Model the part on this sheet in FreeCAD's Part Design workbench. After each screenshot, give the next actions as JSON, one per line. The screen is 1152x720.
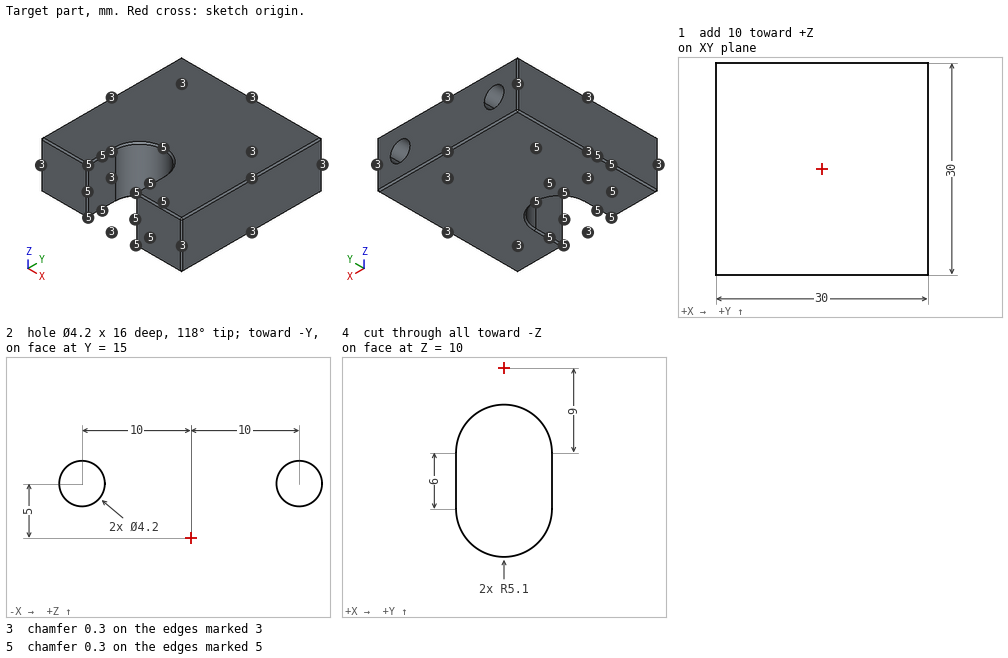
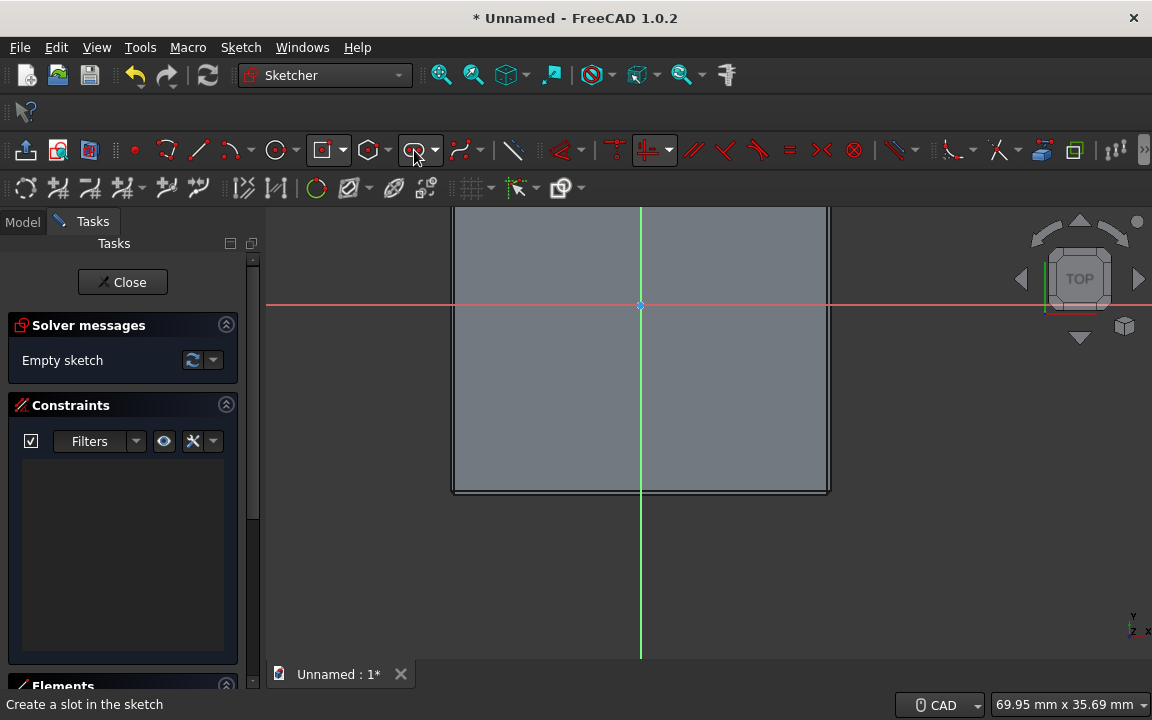
{"action": "left_click", "coordinate": [641, 495]}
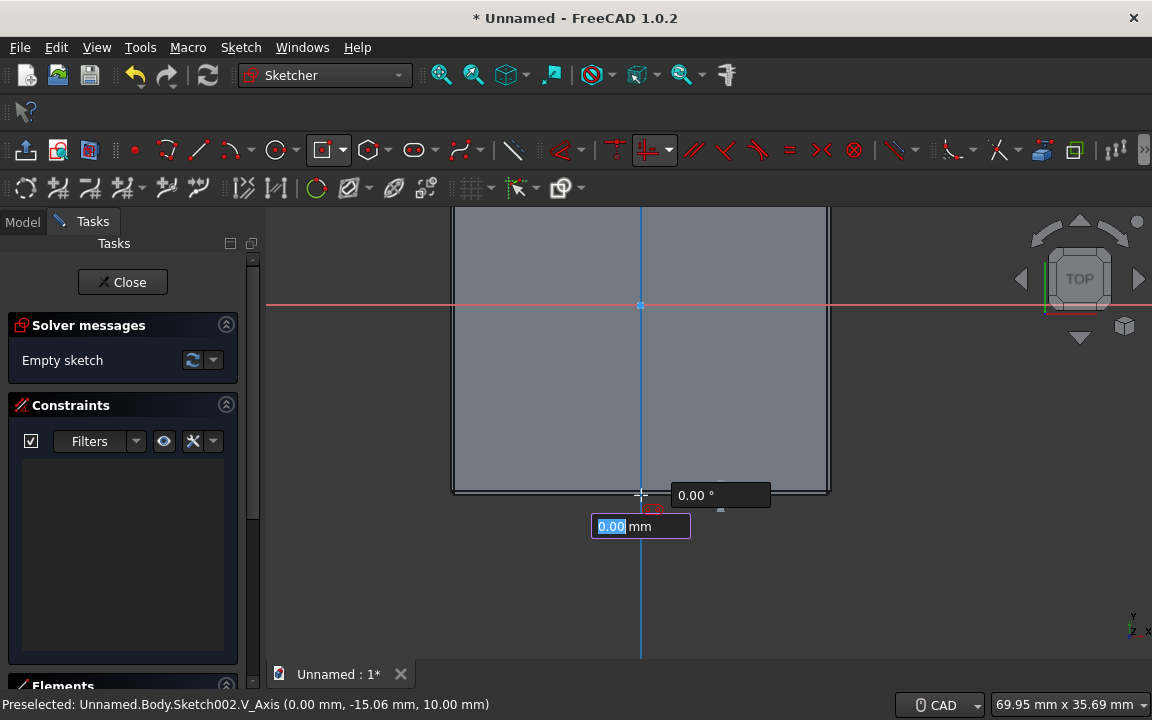
{"action": "left_click", "coordinate": [650, 419]}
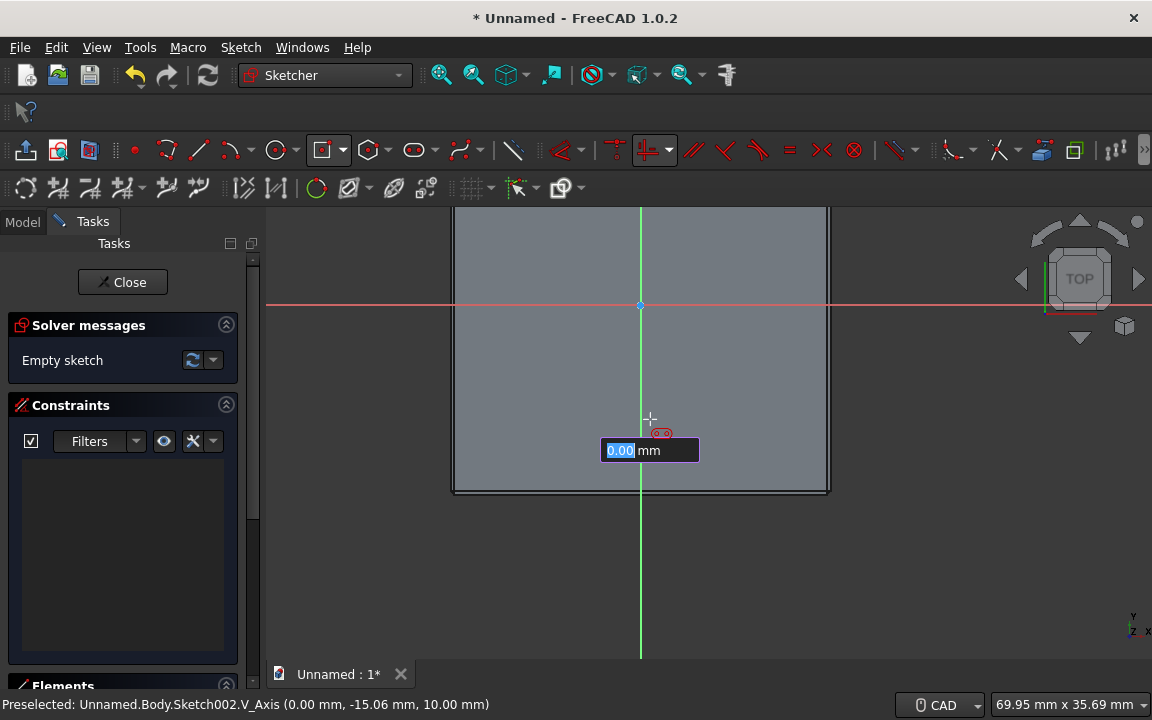
{"action": "left_click", "coordinate": [576, 457]}
{"action": "key", "text": "Escape"}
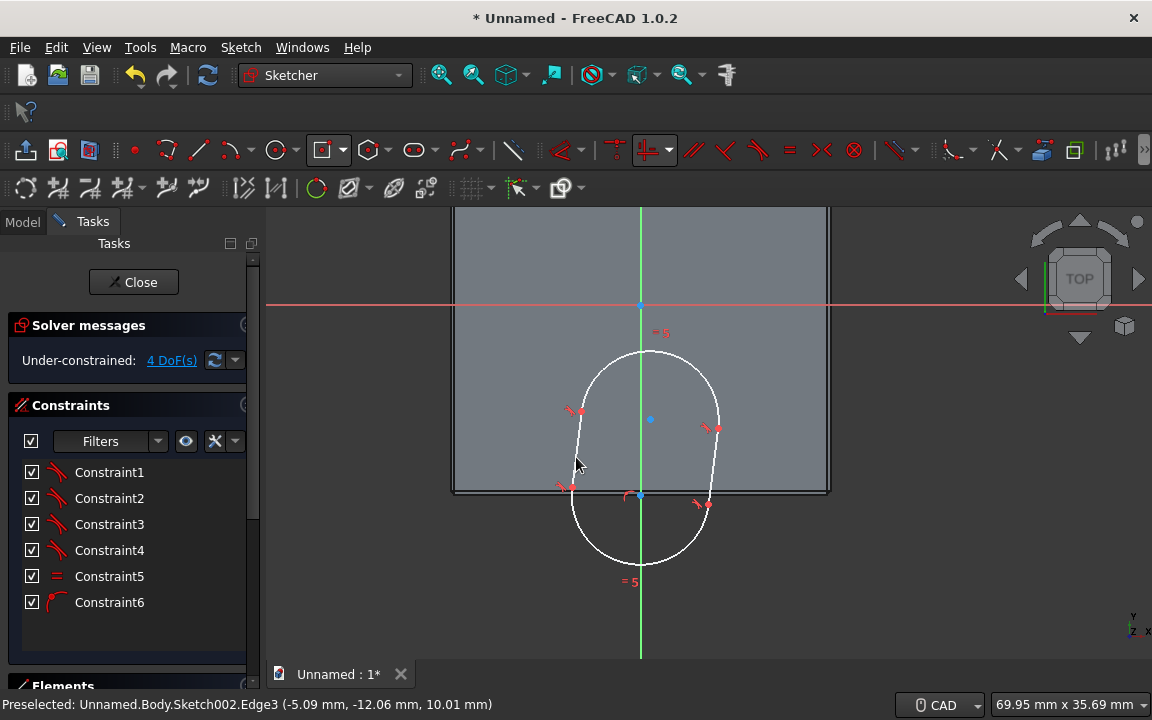
{"action": "left_click", "coordinate": [575, 465]}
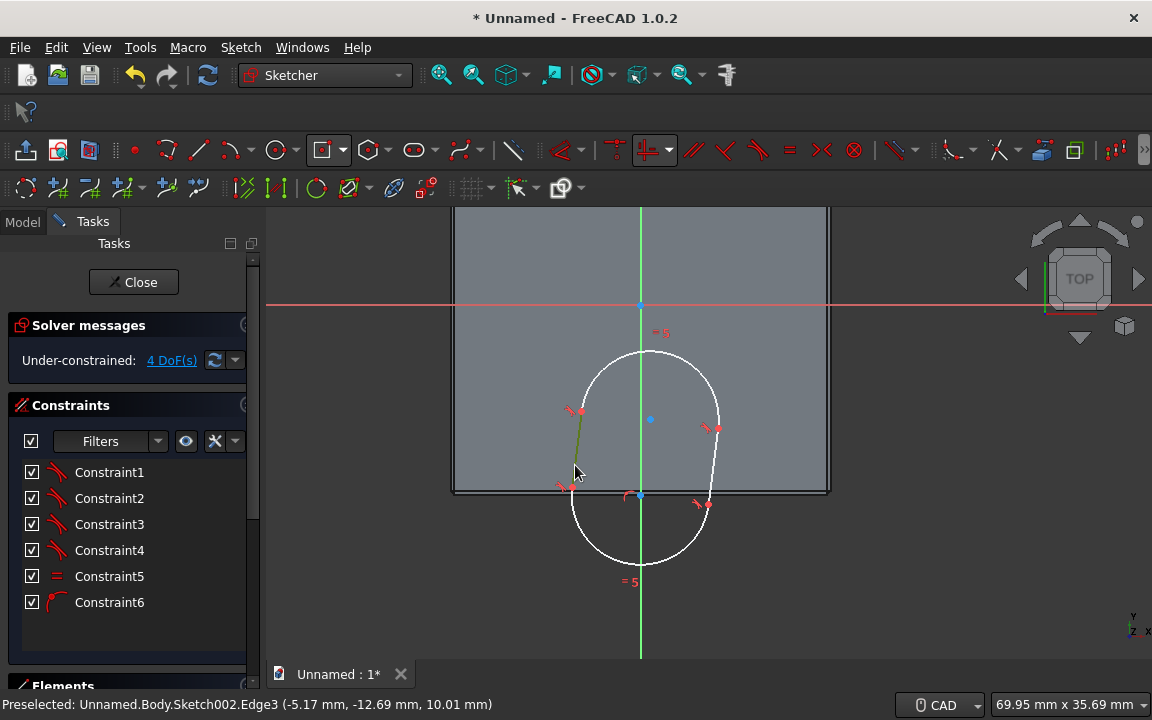
{"action": "left_click", "coordinate": [672, 150]}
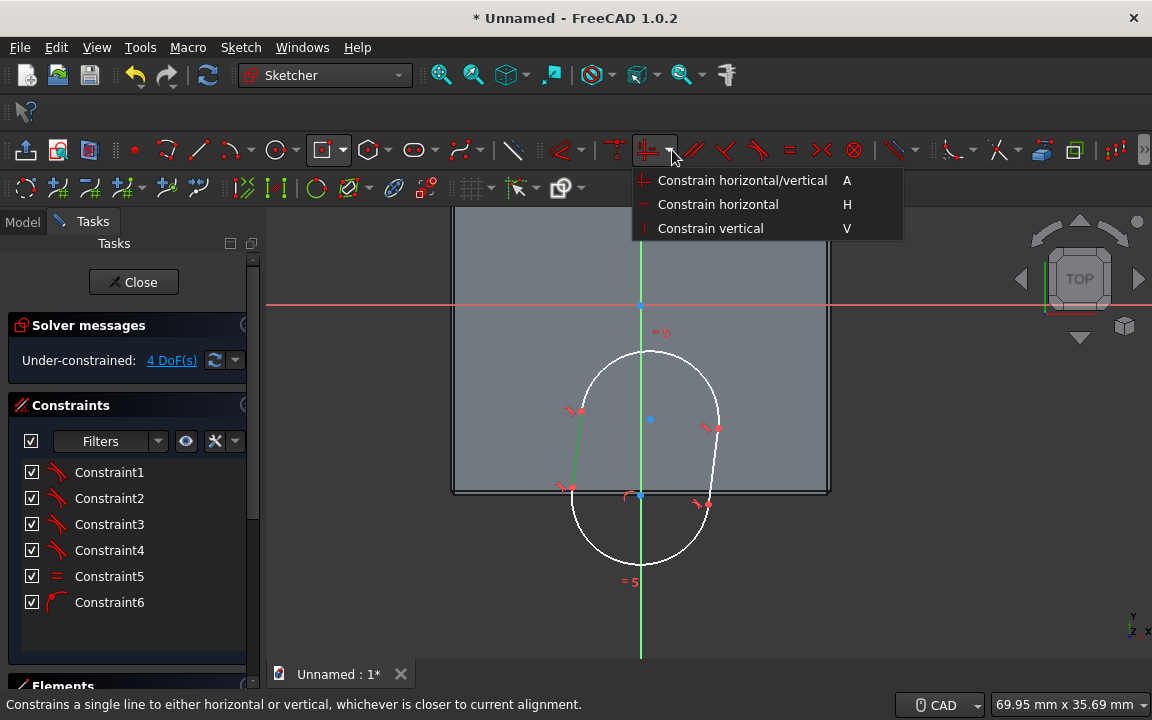
{"action": "left_click", "coordinate": [768, 228]}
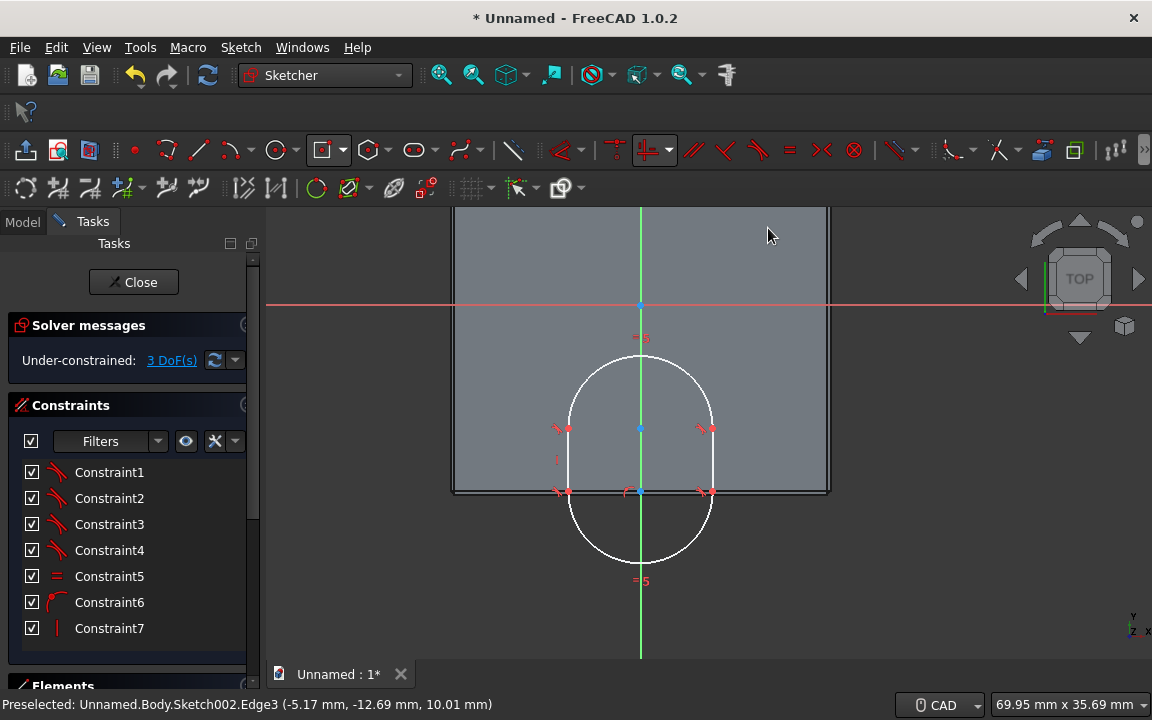
{"action": "left_click", "coordinate": [560, 150]}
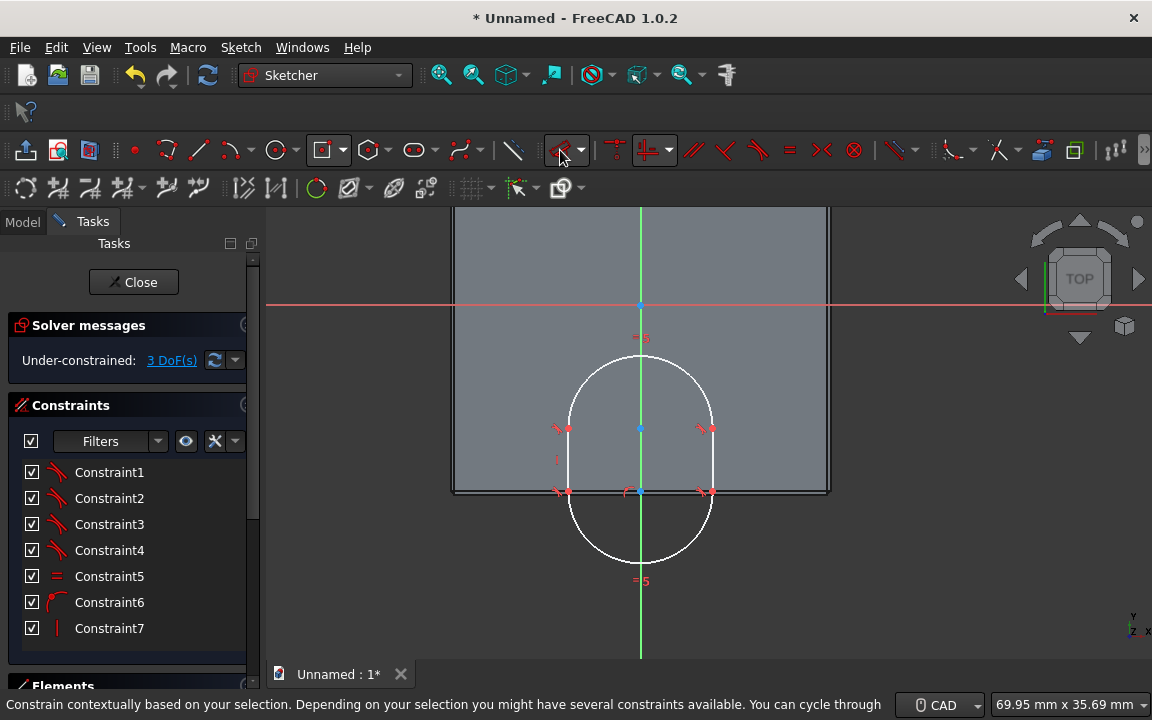
{"action": "left_click", "coordinate": [598, 550]}
{"action": "left_click", "coordinate": [579, 576]}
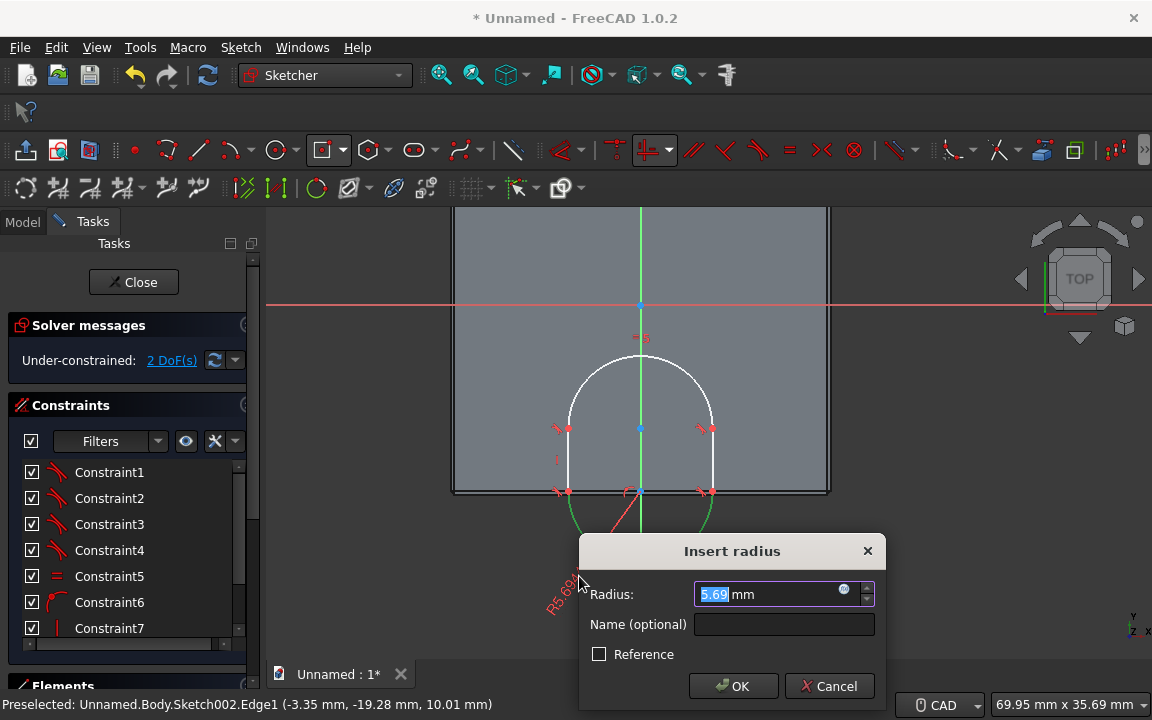
{"action": "type", "text": "5.1"}
{"action": "key", "text": "Return"}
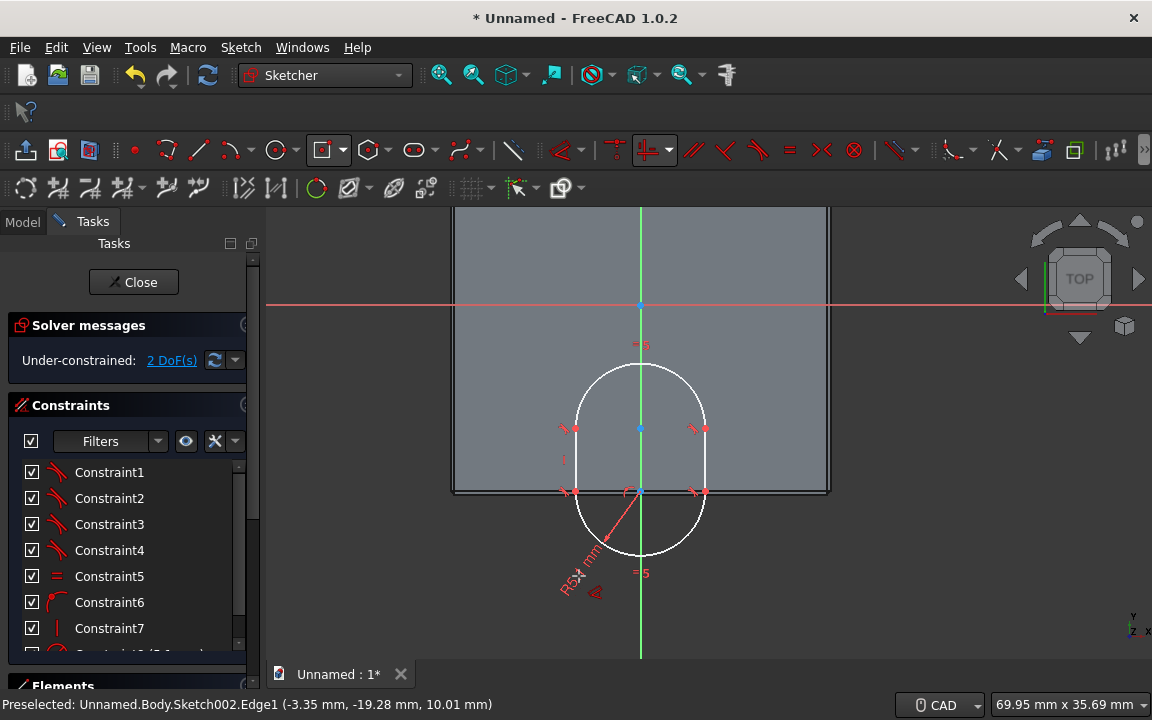
{"action": "left_click", "coordinate": [576, 472]}
{"action": "left_click", "coordinate": [542, 460]}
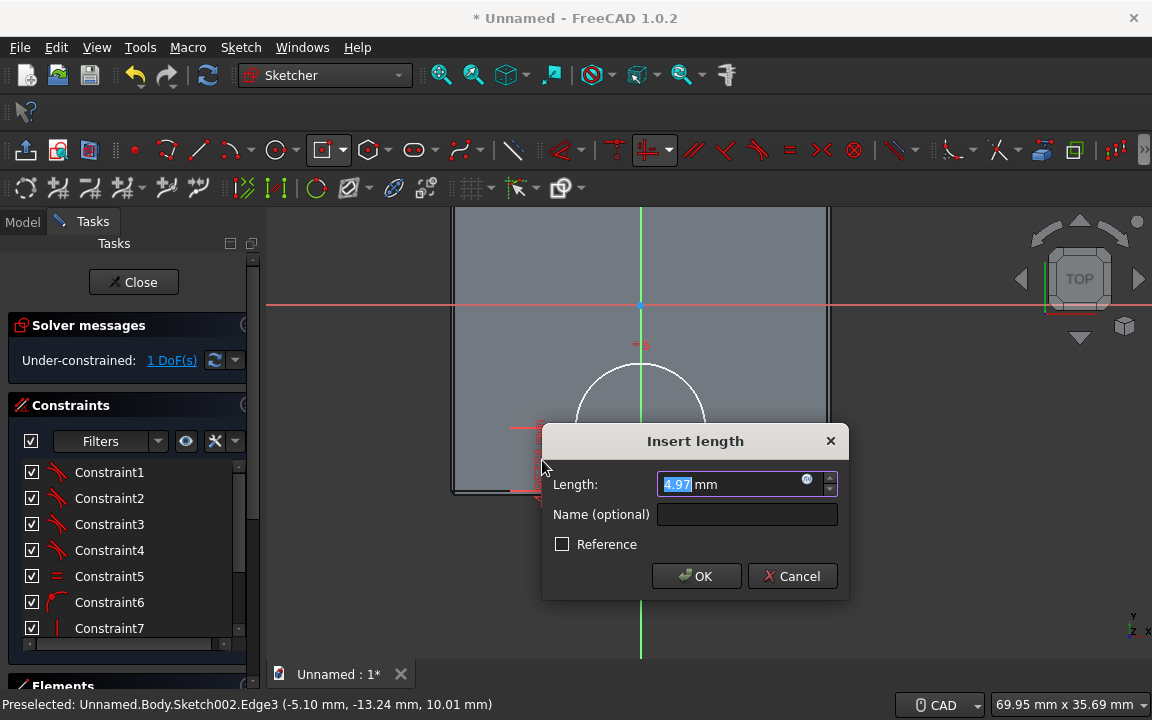
{"action": "type", "text": "6"}
{"action": "key", "text": "Return"}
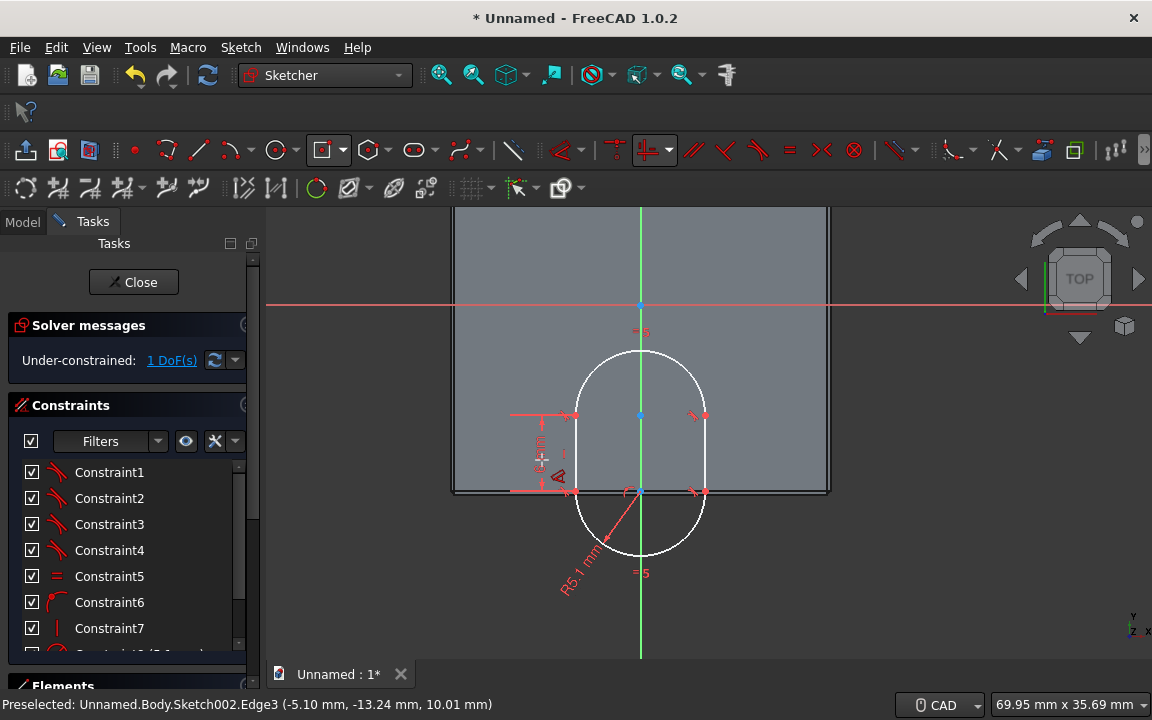
{"action": "left_click", "coordinate": [705, 415]}
{"action": "left_click", "coordinate": [739, 360]}